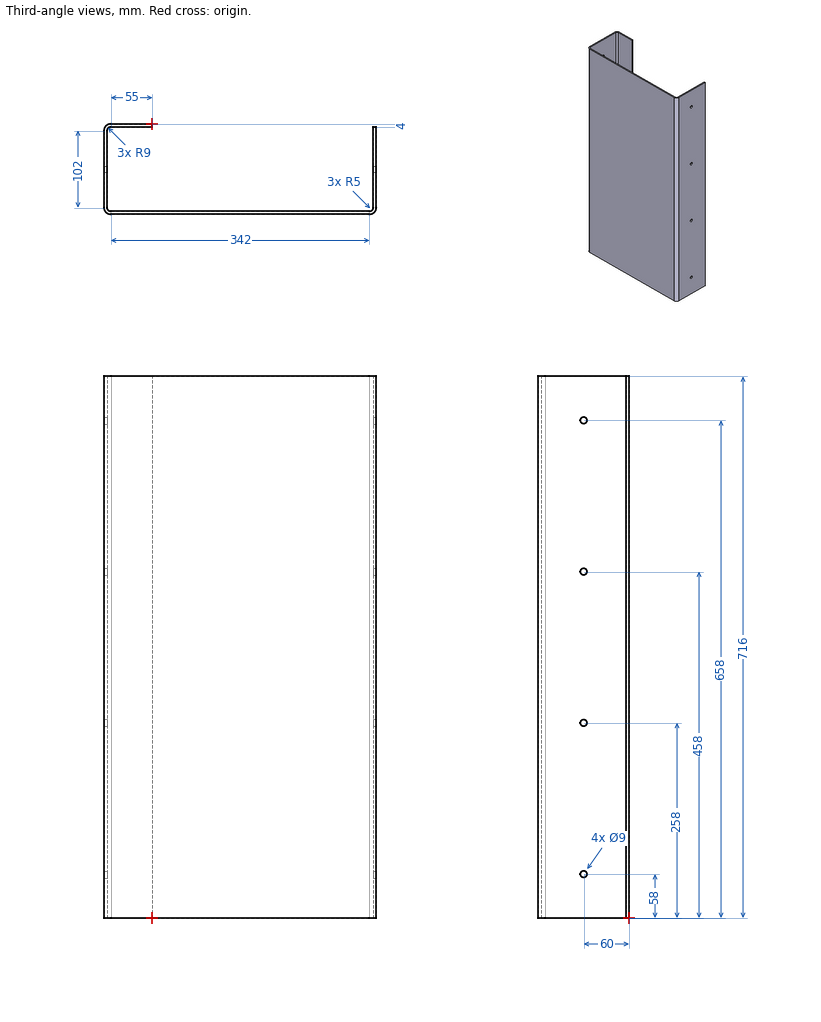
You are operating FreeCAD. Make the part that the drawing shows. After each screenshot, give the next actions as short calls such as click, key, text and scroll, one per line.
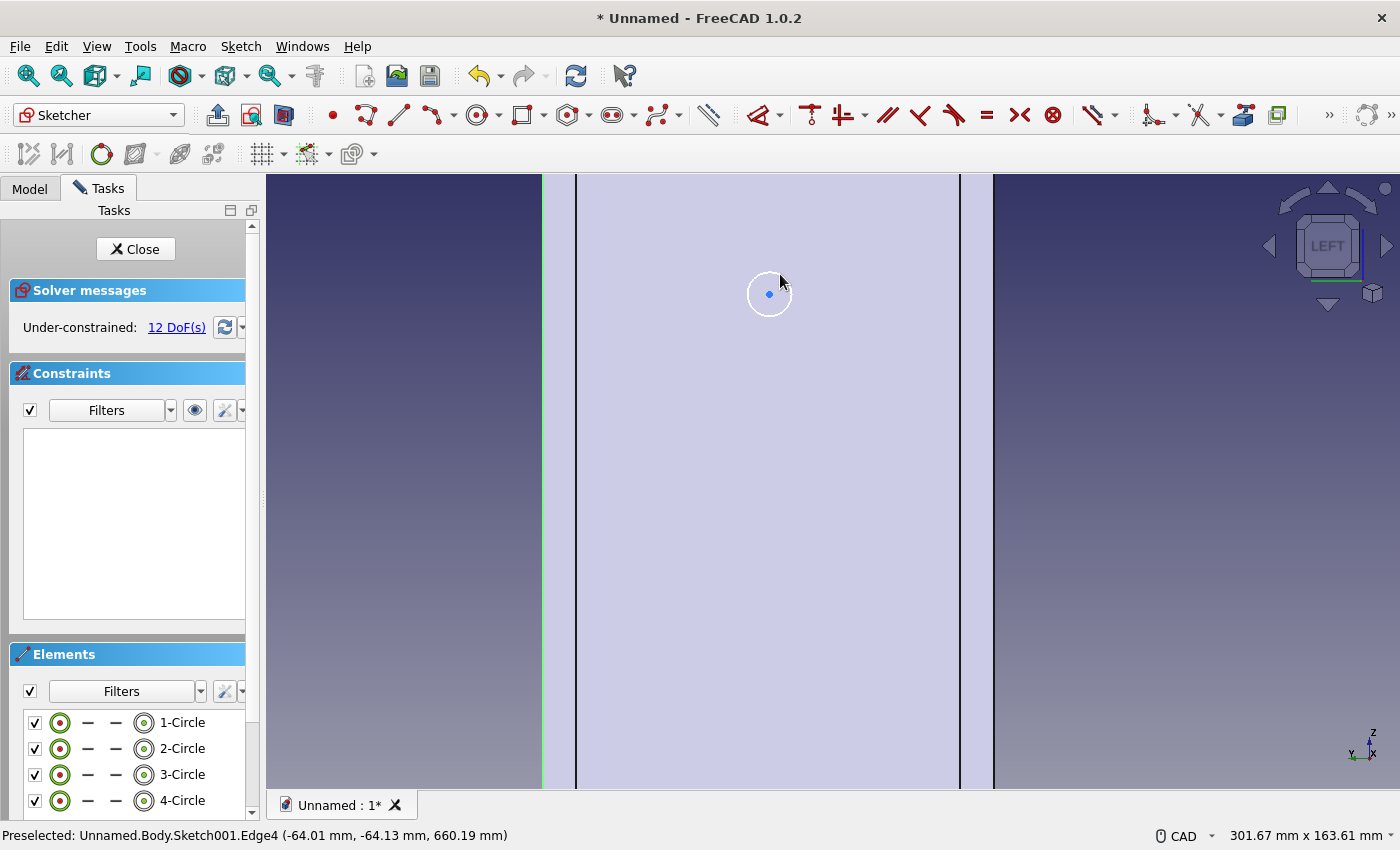
scroll(784, 277, down, 9)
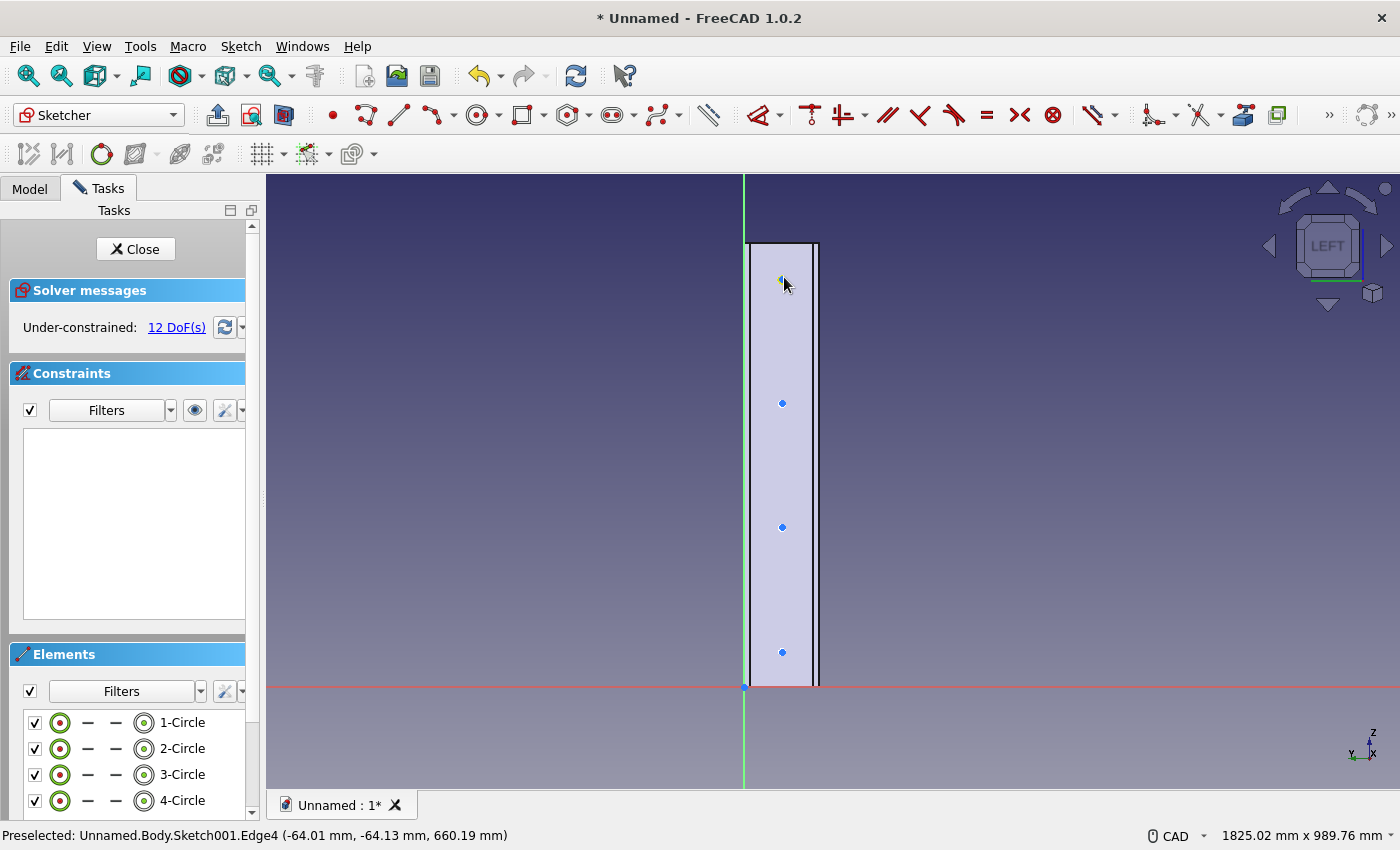
scroll(784, 650, up, 8)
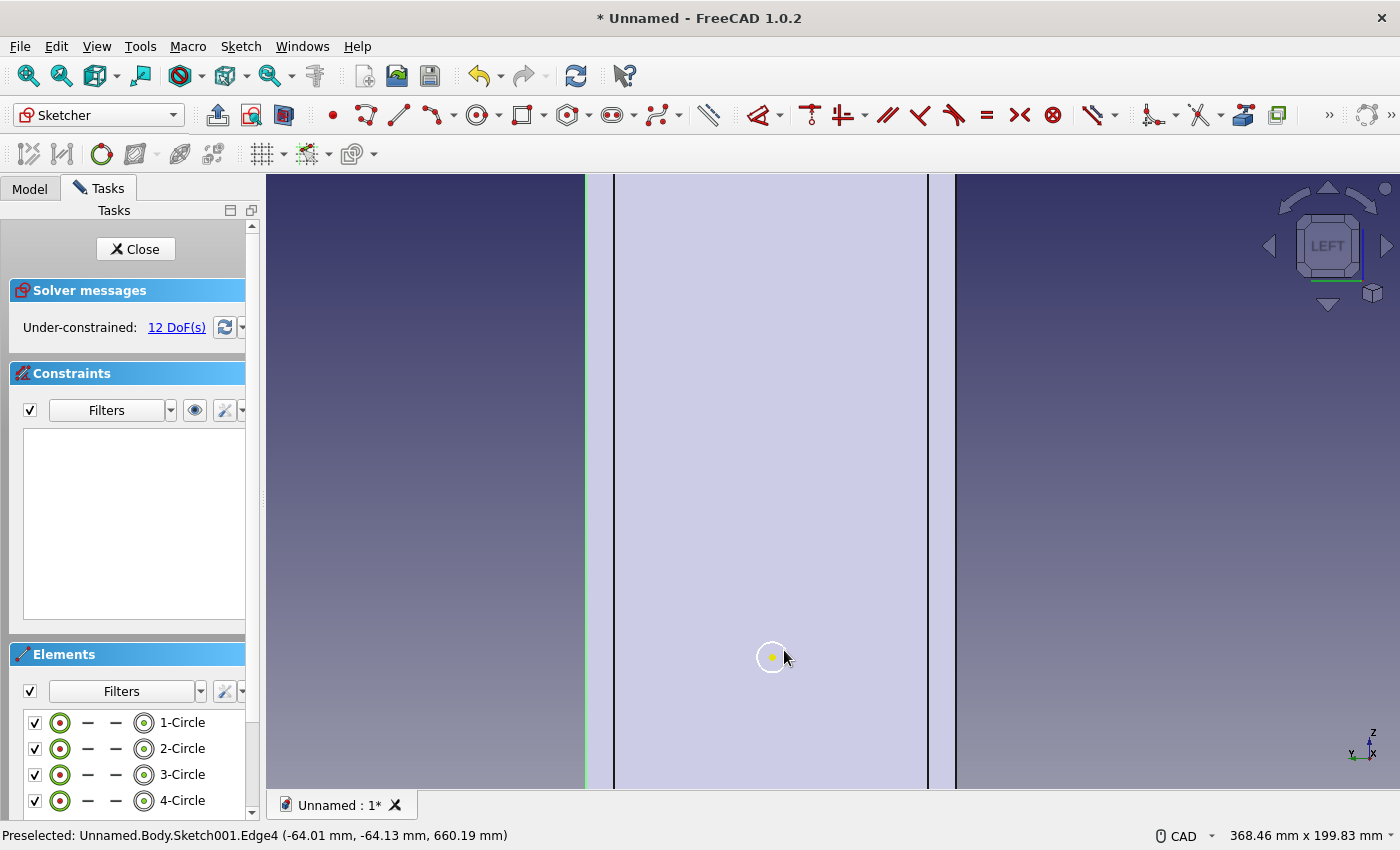
click(783, 647)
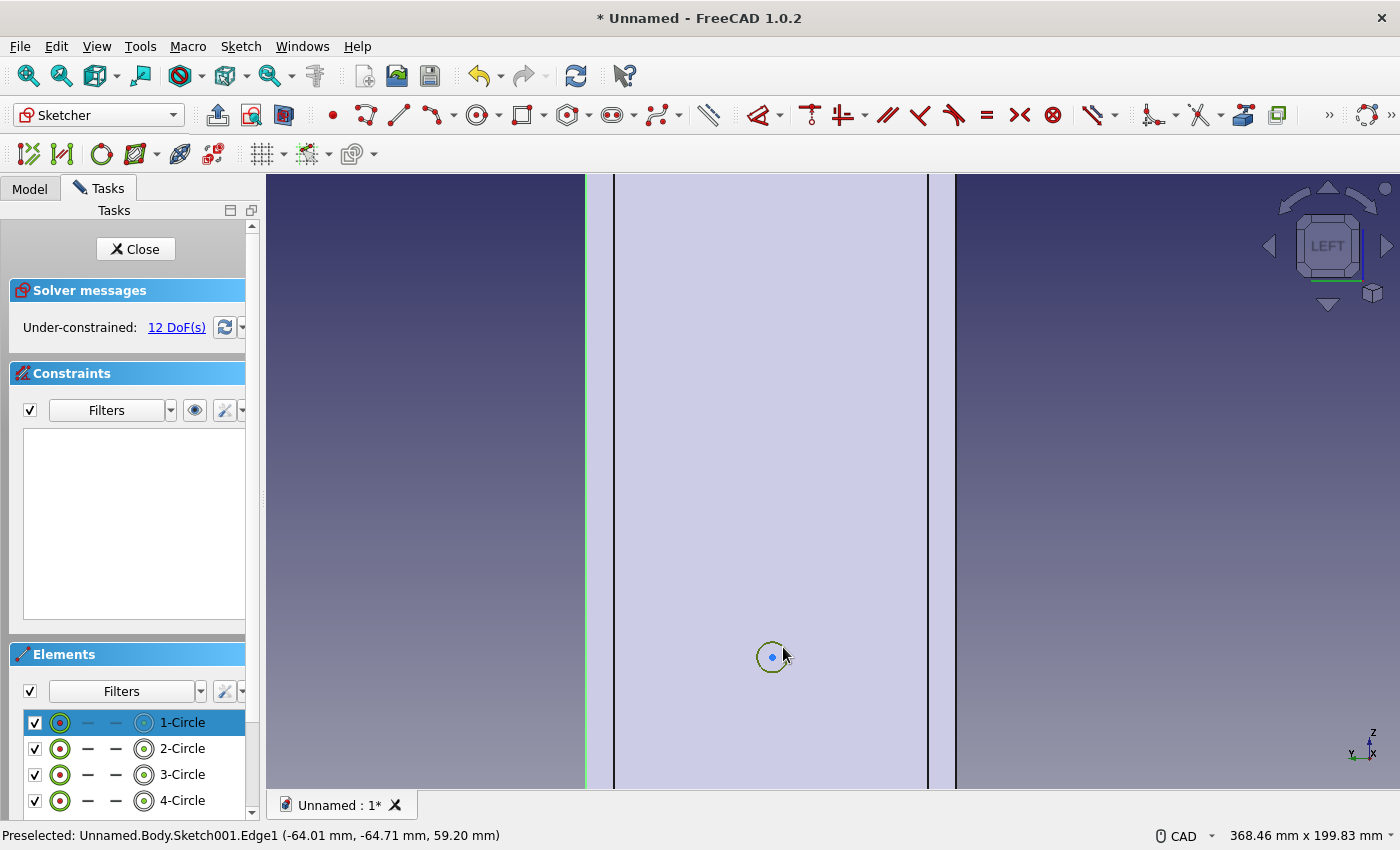
scroll(784, 651, down, 8)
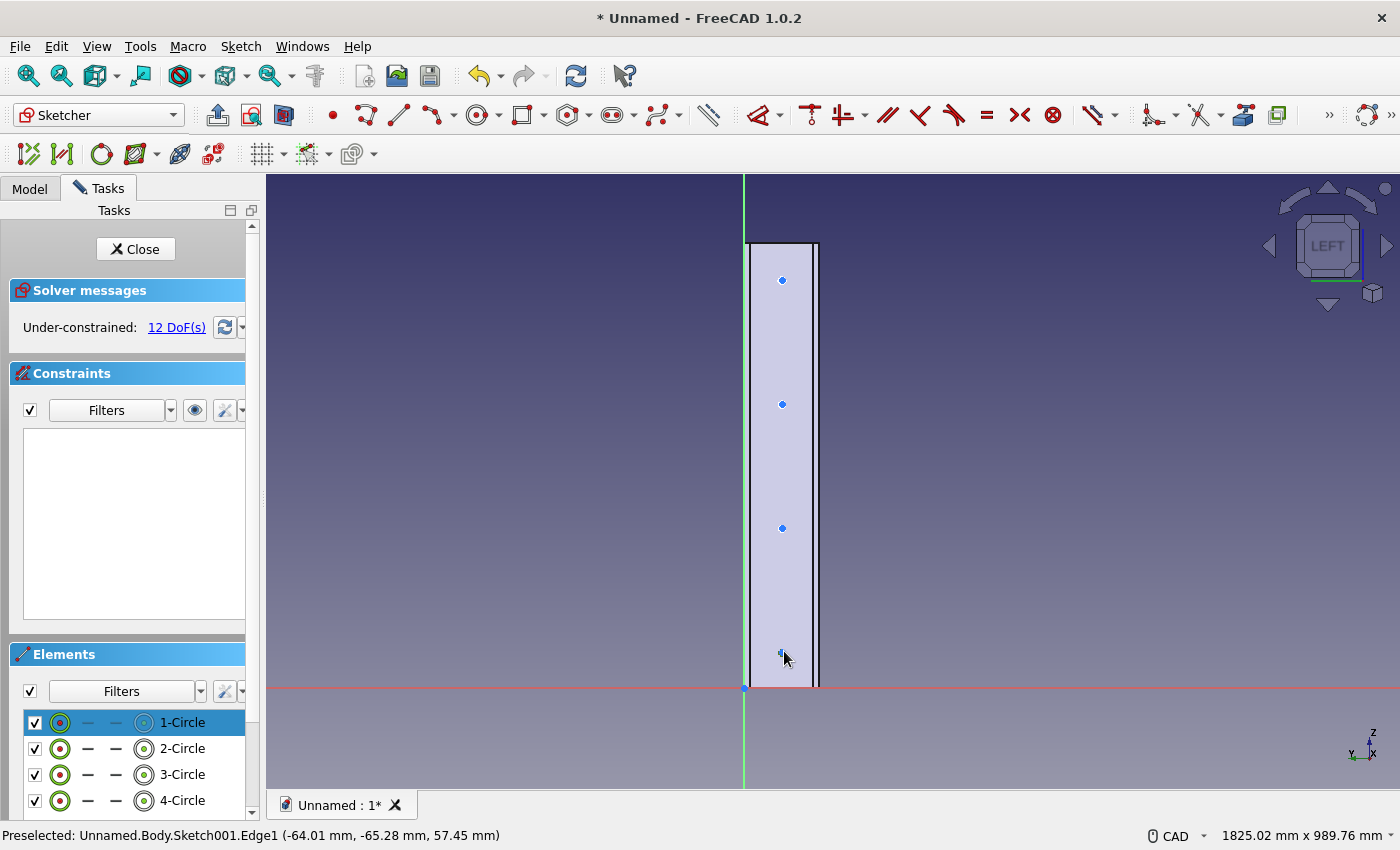
scroll(784, 527, up, 8)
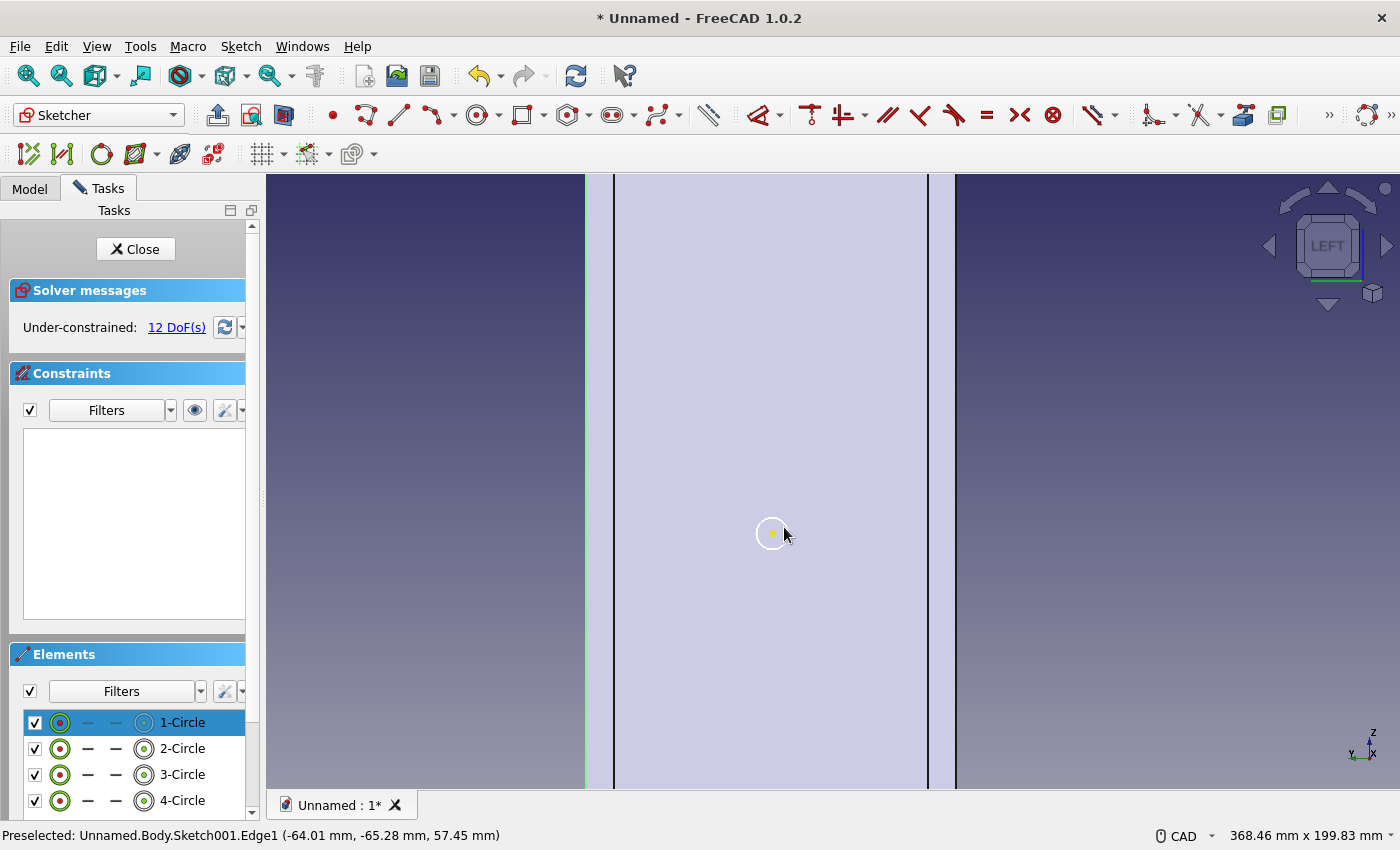
click(783, 522)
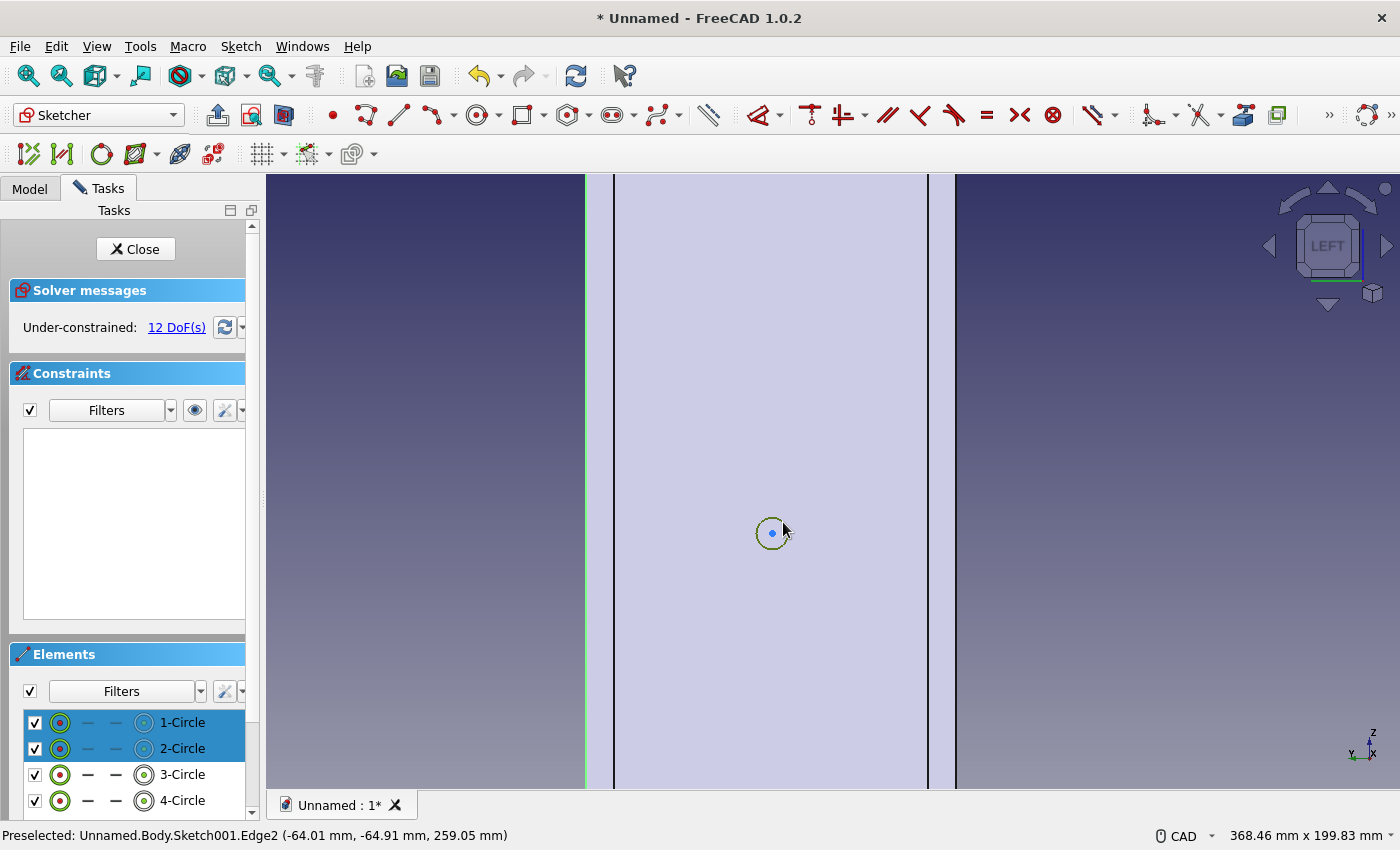
scroll(784, 526, down, 8)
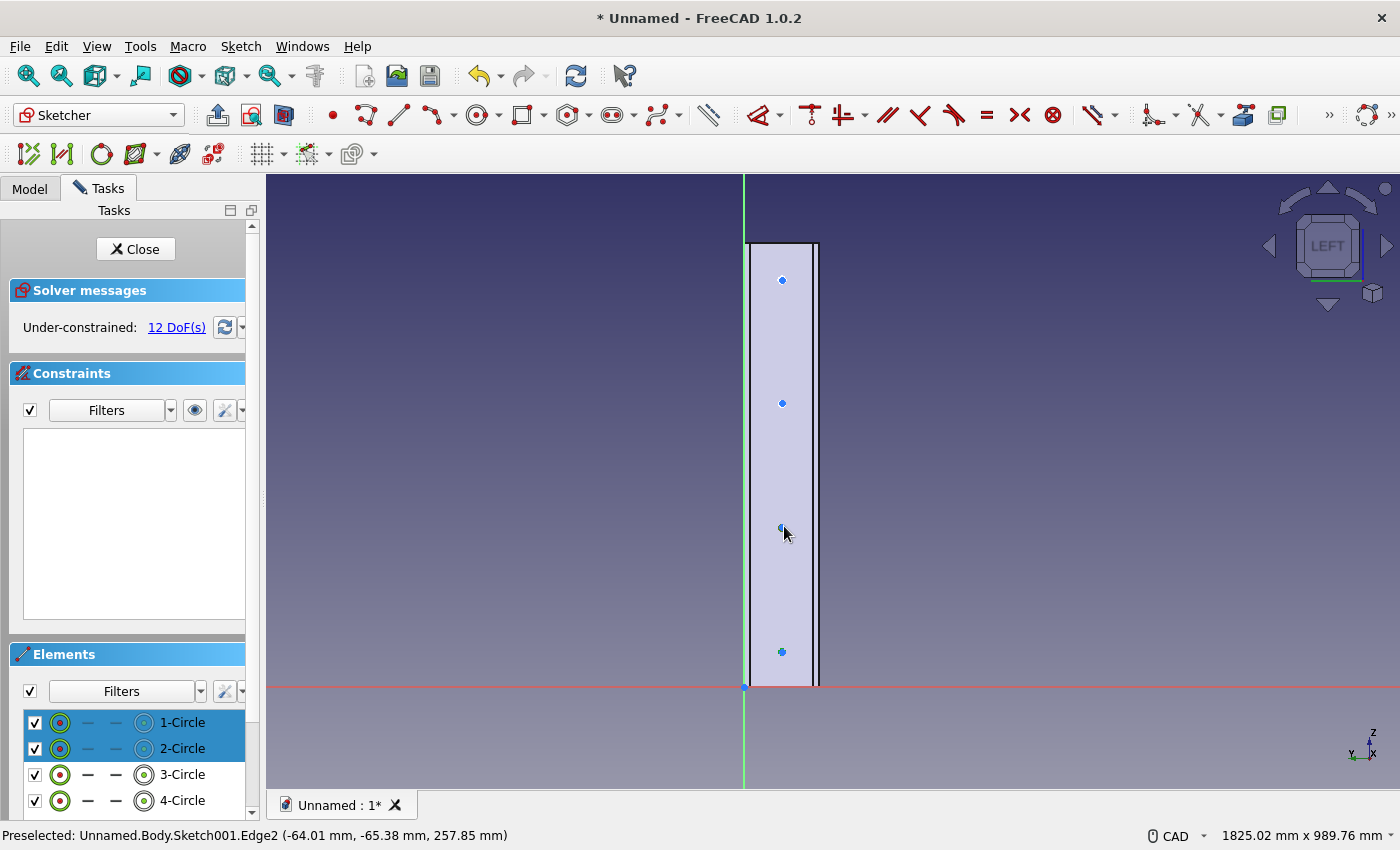
scroll(784, 402, up, 7)